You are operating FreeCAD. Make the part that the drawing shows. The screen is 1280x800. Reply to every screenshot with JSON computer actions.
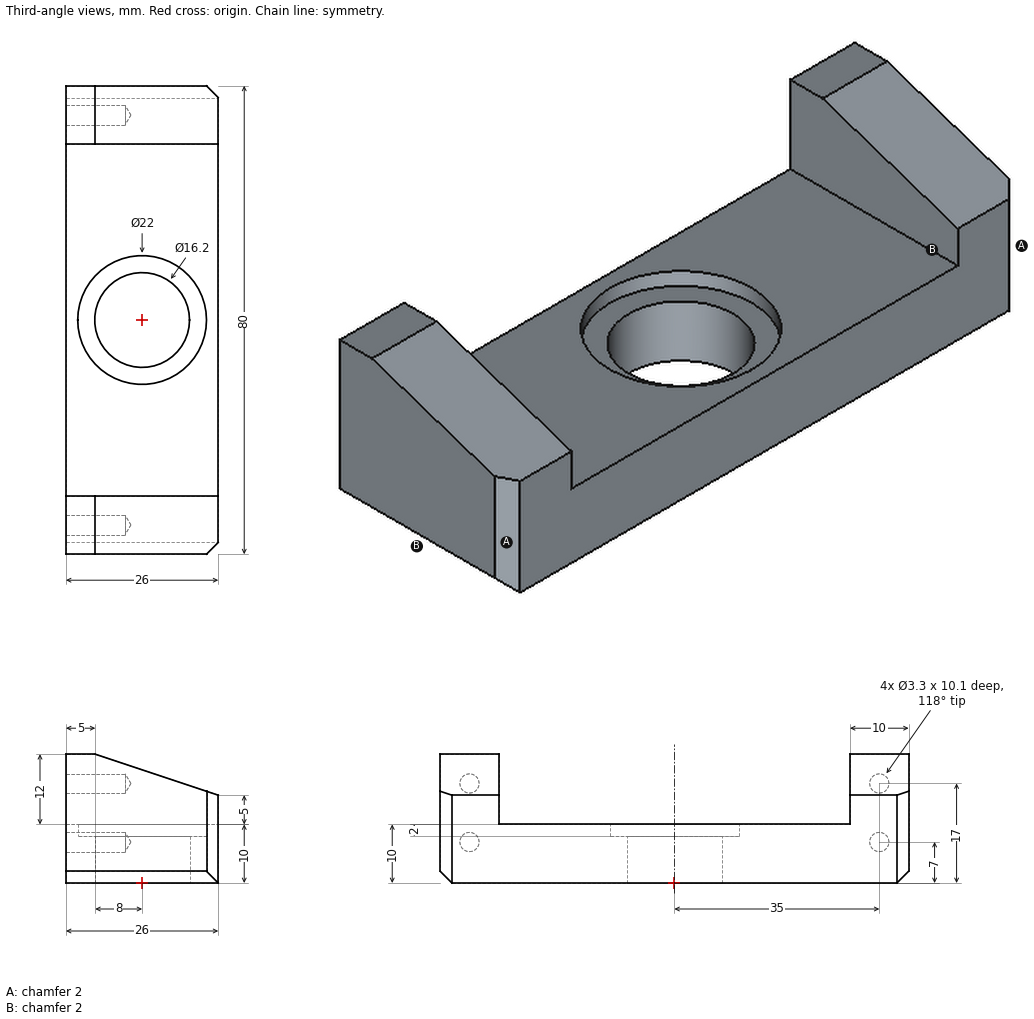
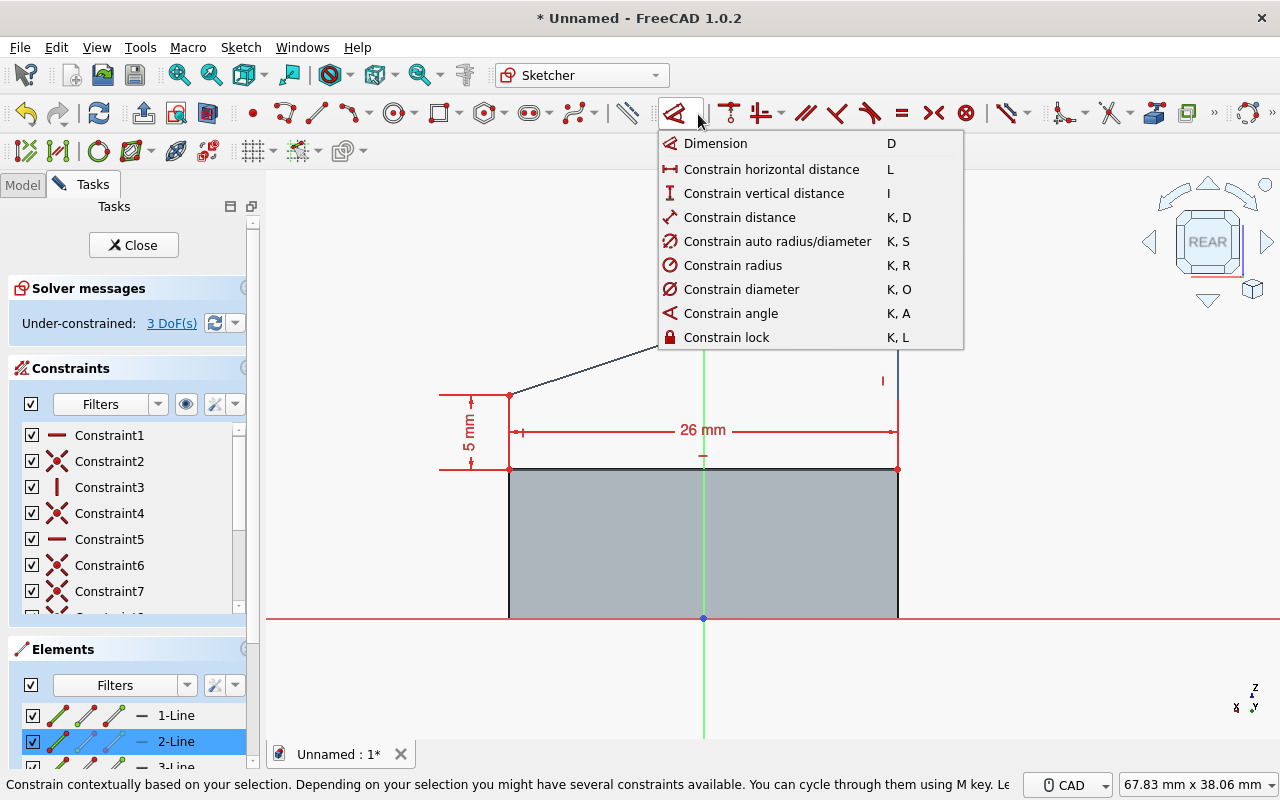
{"action": "left_click", "coordinate": [811, 193]}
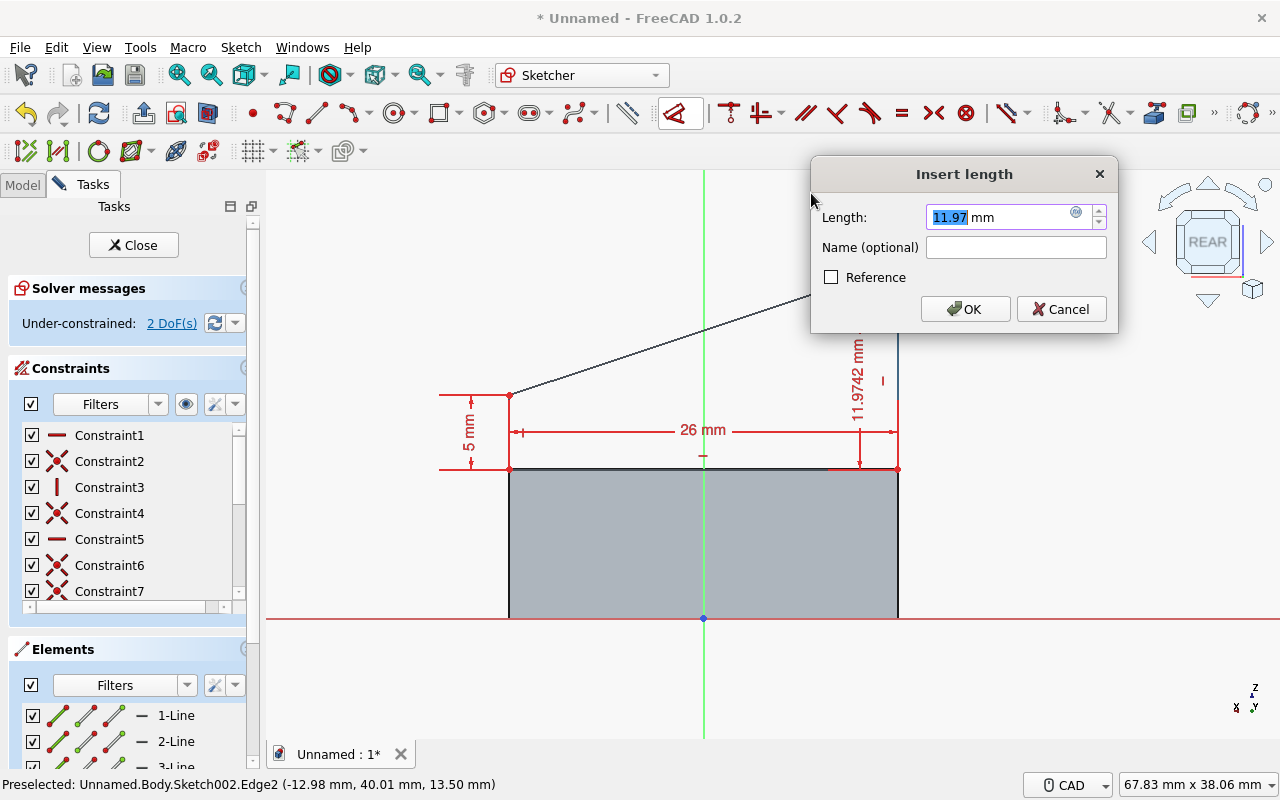
{"action": "type", "text": "12"}
{"action": "key", "text": "Return"}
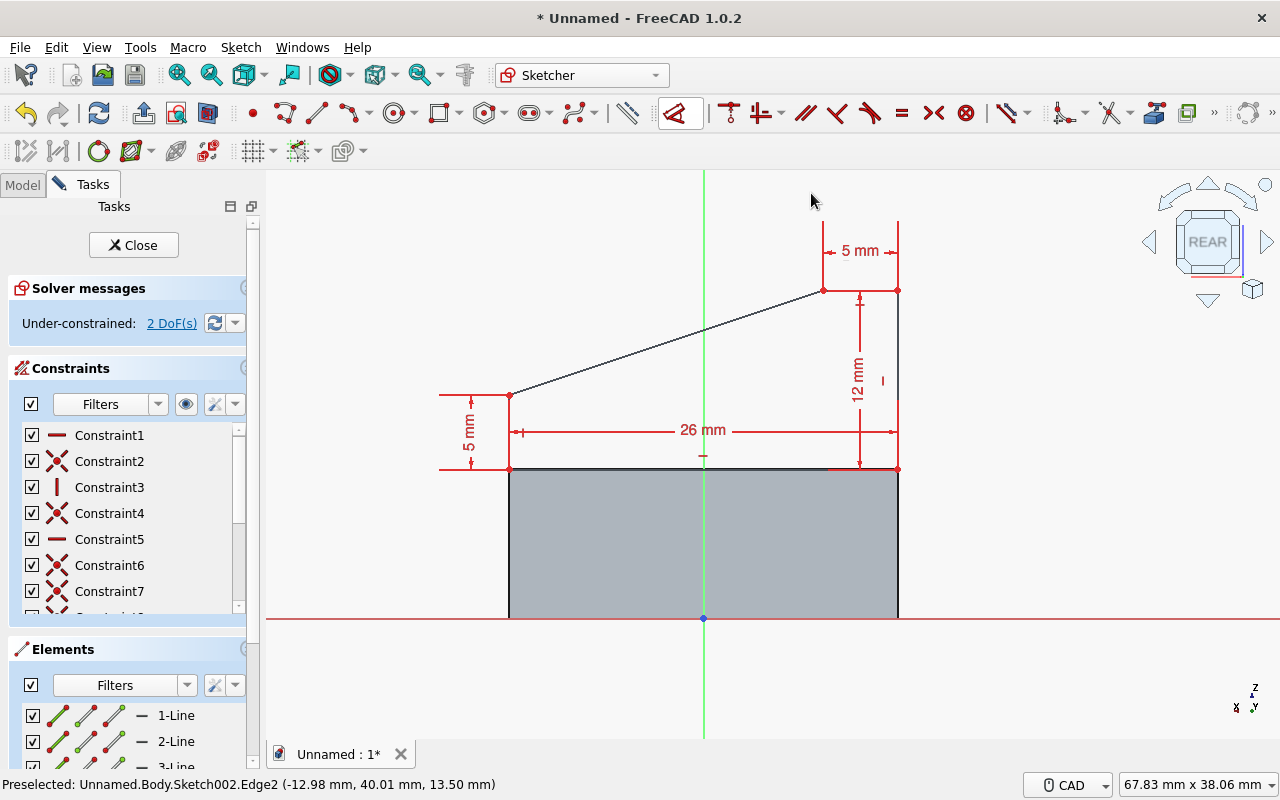
{"action": "left_click", "coordinate": [823, 291]}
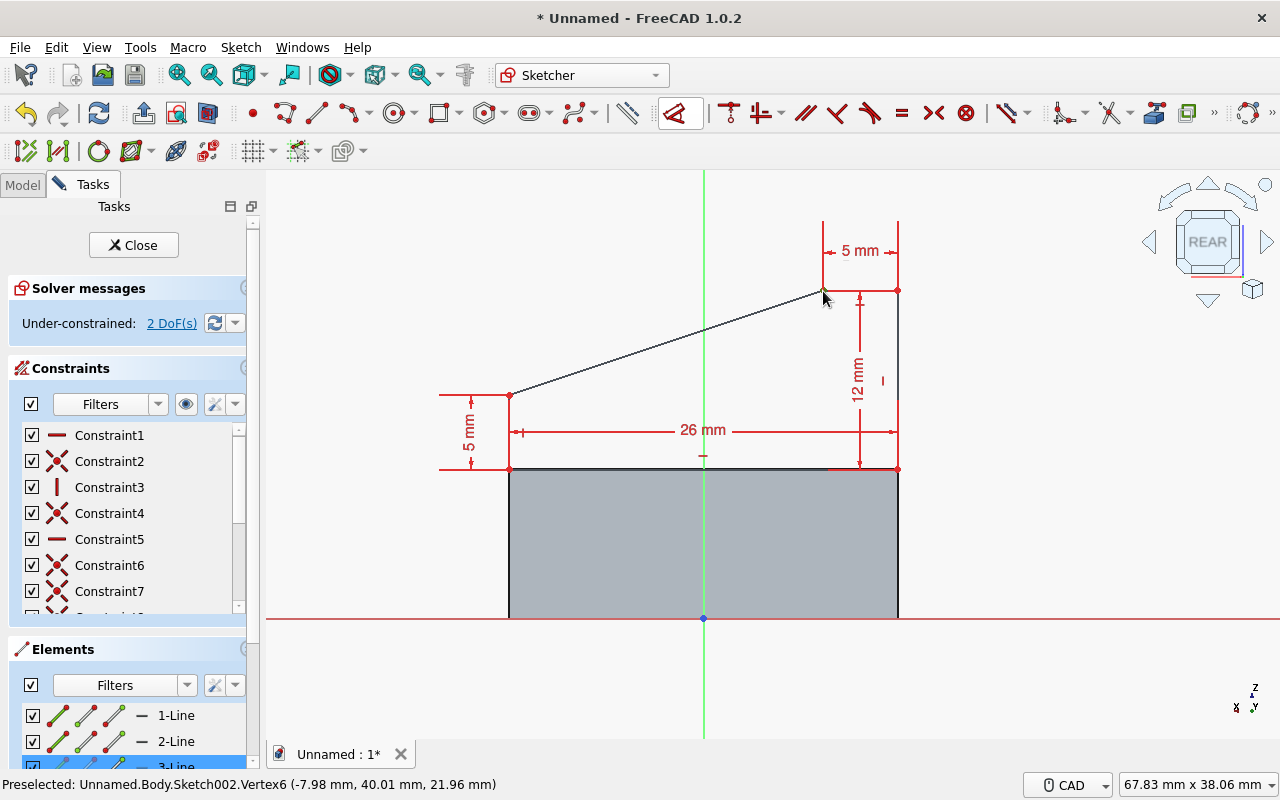
{"action": "left_click", "coordinate": [698, 114]}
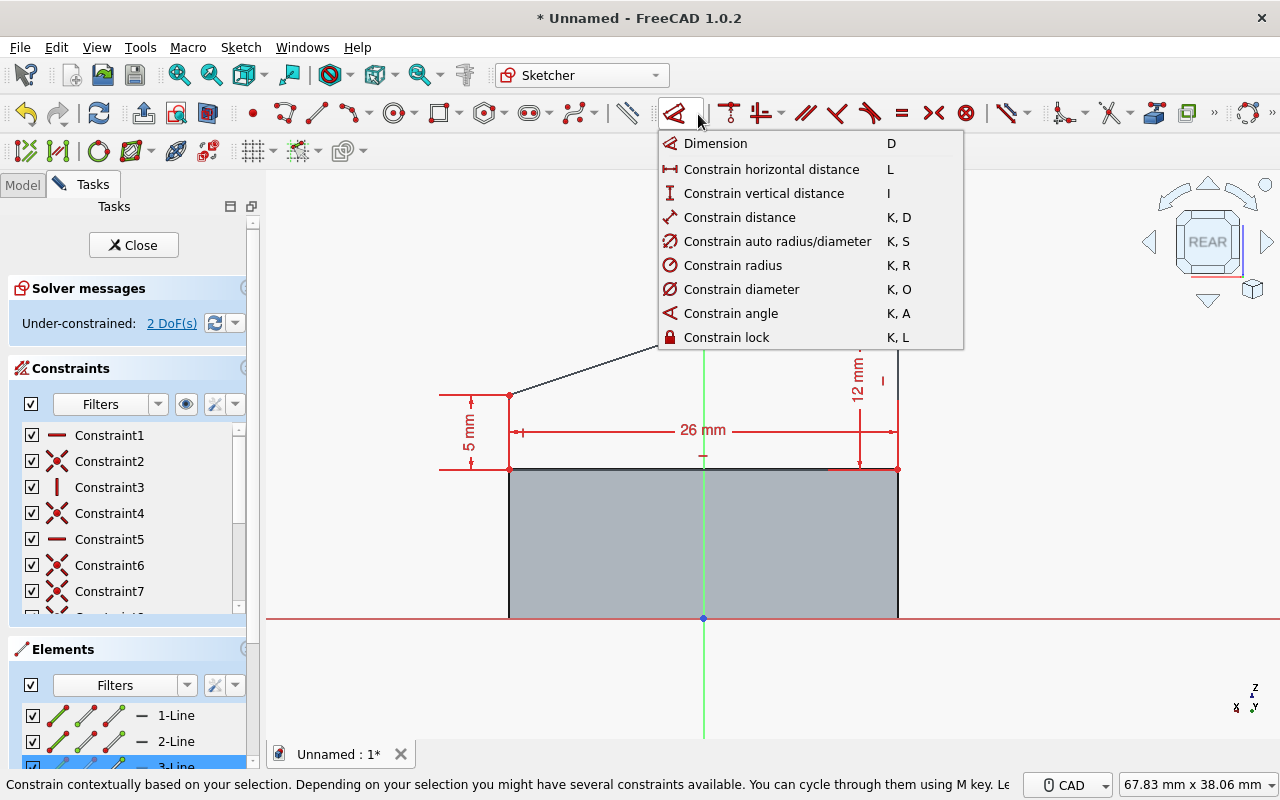
{"action": "left_click", "coordinate": [811, 169]}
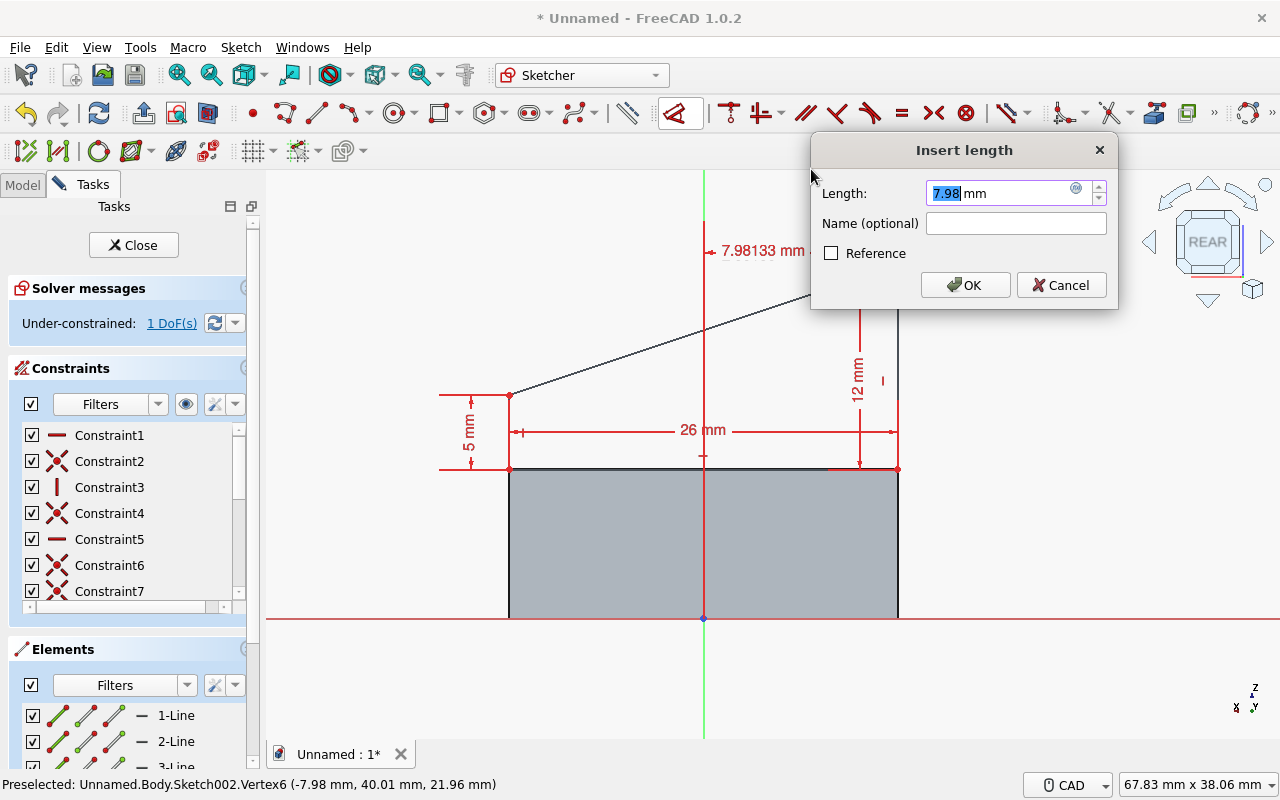
{"action": "type", "text": "8"}
{"action": "key", "text": "Return"}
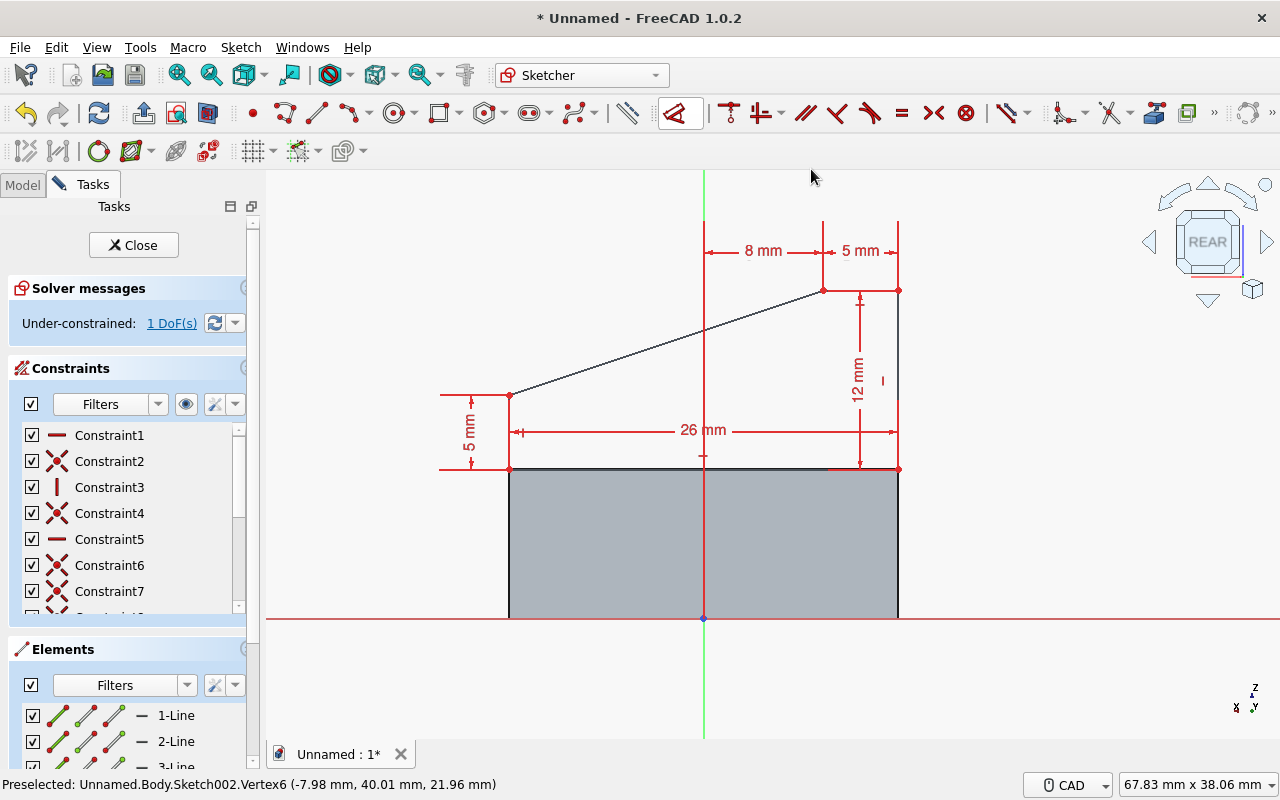
{"action": "left_click", "coordinate": [509, 470]}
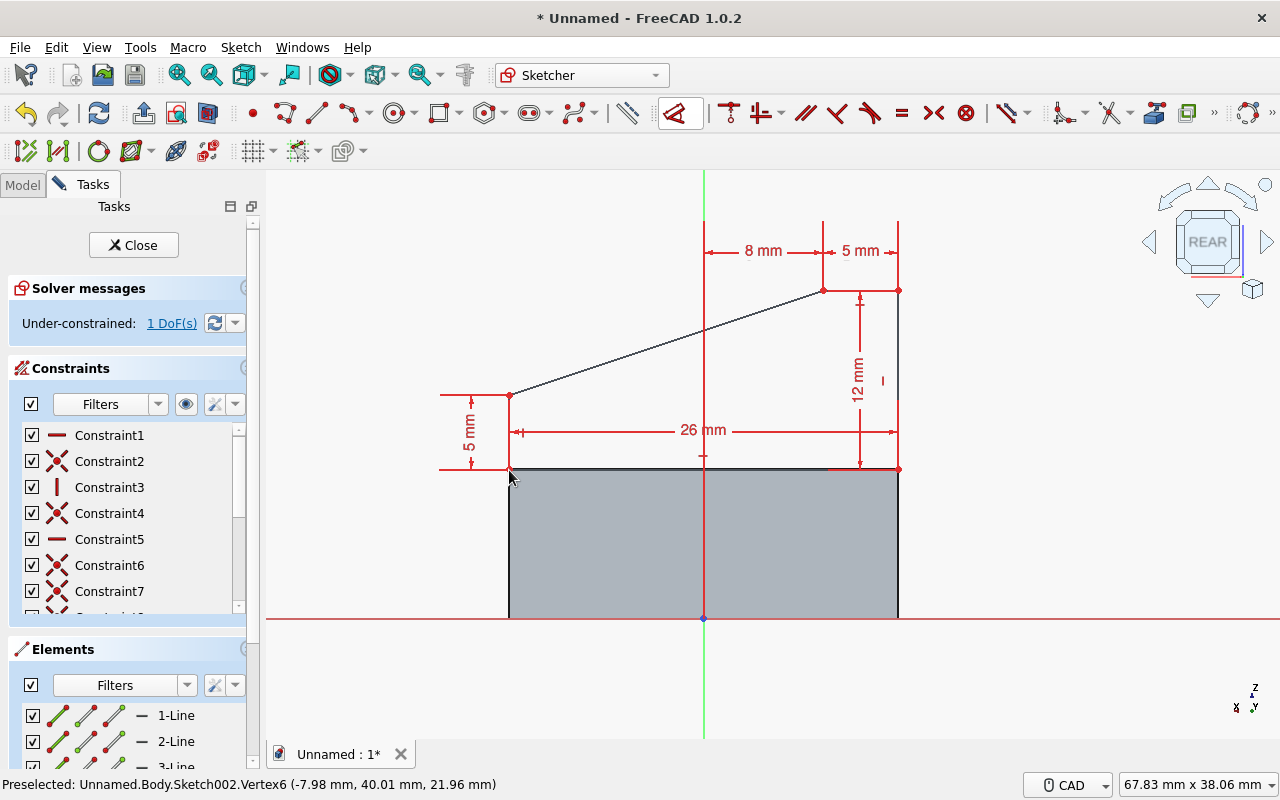
{"action": "left_click", "coordinate": [698, 114]}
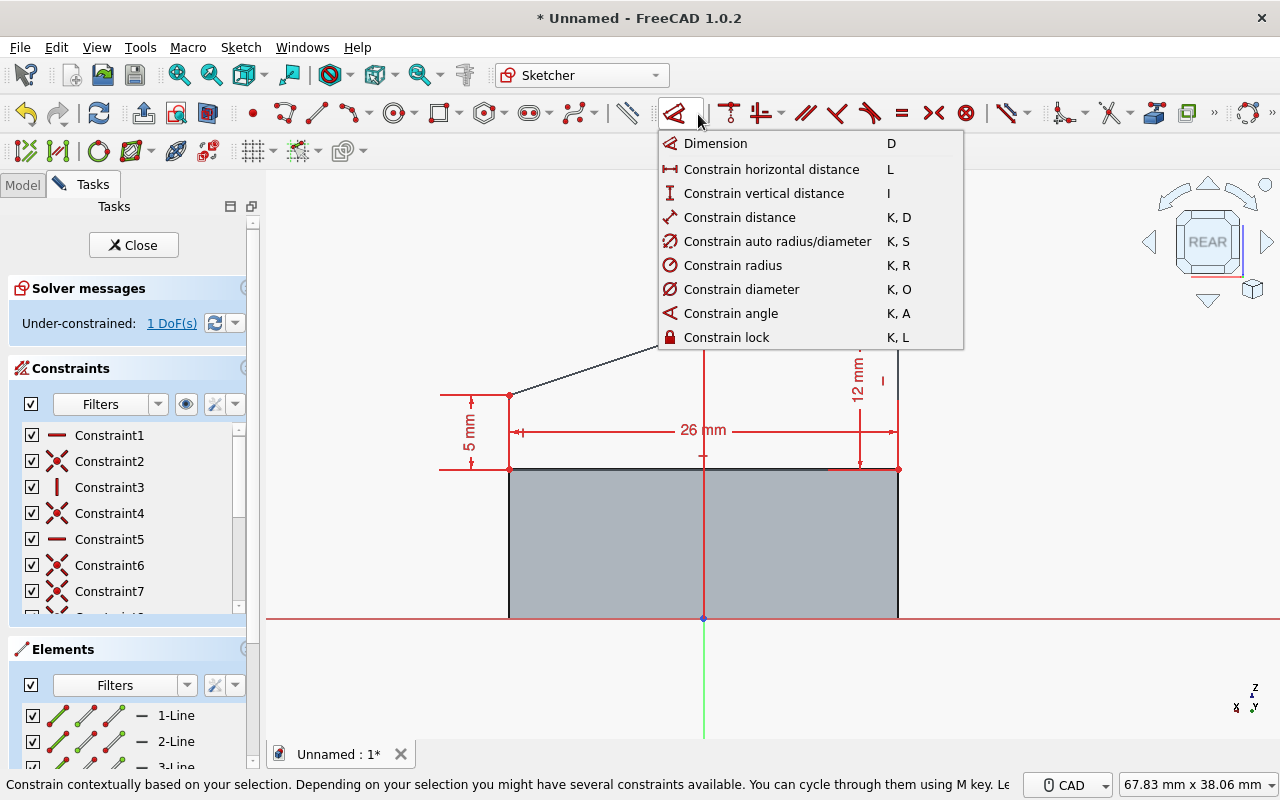
{"action": "left_click", "coordinate": [811, 193]}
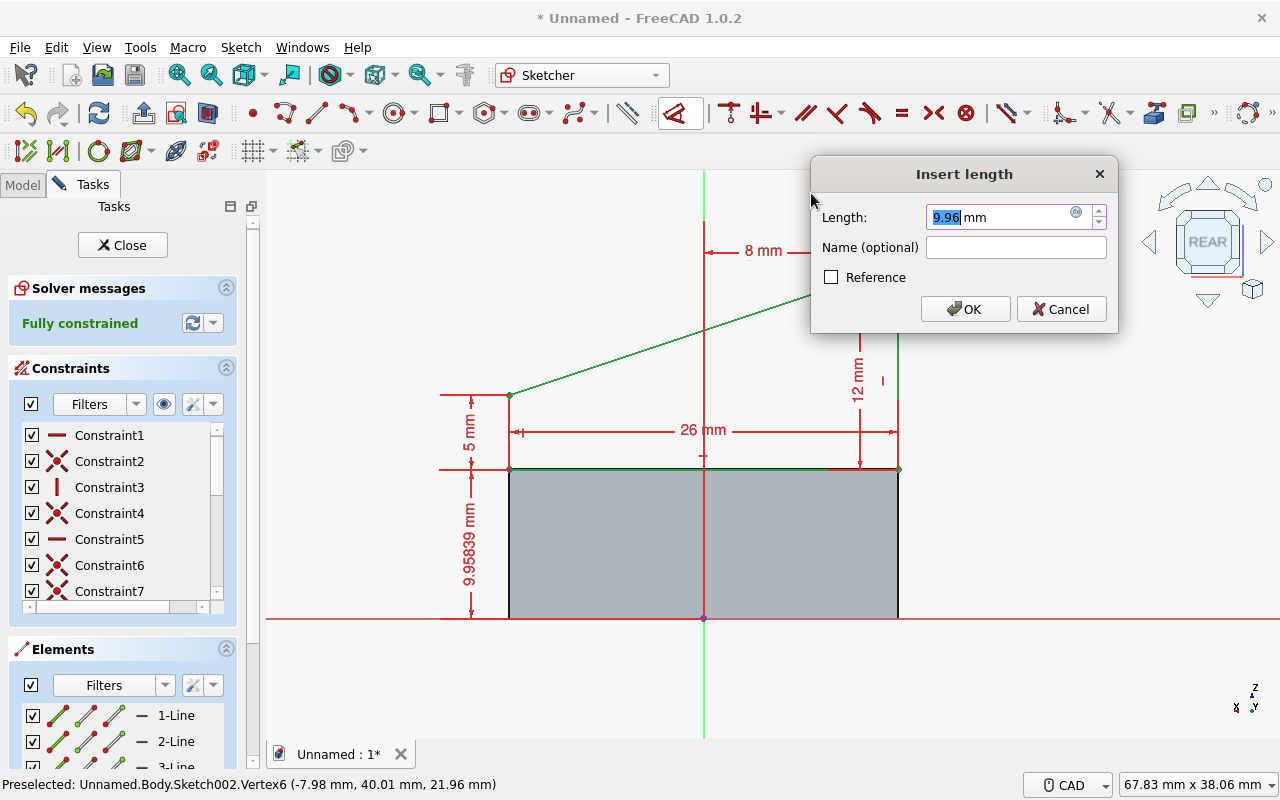
{"action": "type", "text": "10"}
{"action": "key", "text": "Return"}